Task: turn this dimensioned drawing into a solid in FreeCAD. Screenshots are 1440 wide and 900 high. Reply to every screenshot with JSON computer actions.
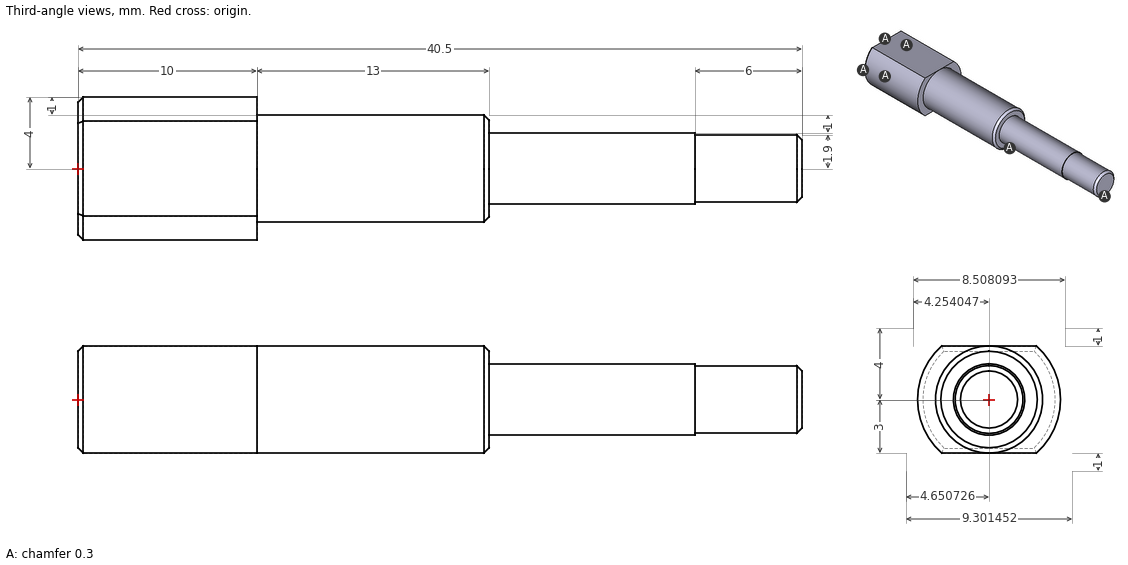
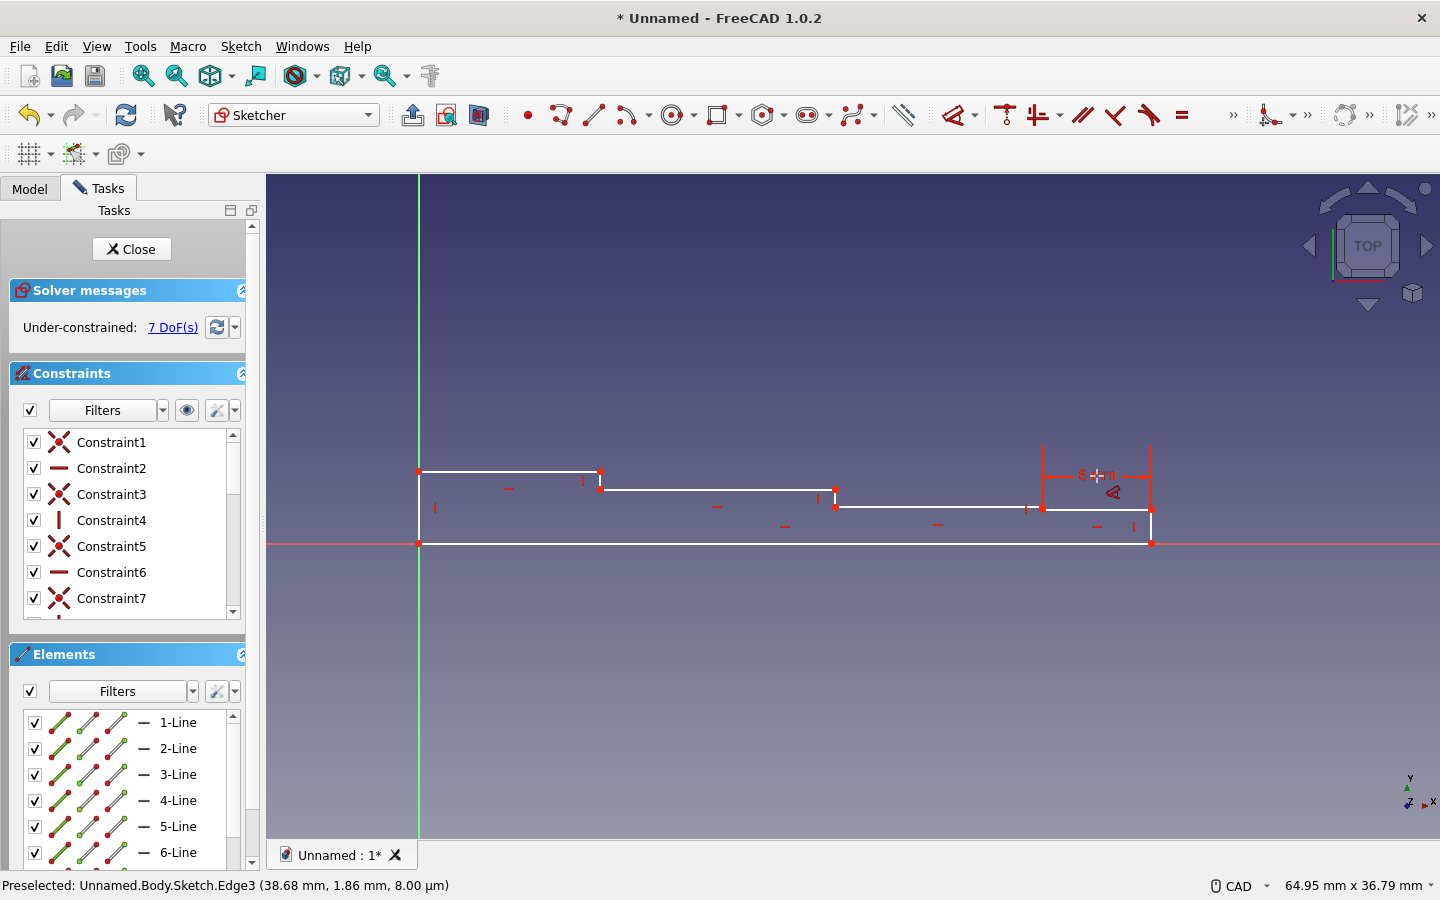
{"action": "scroll", "coordinate": [835, 499], "scroll_direction": "up", "scroll_amount": 4}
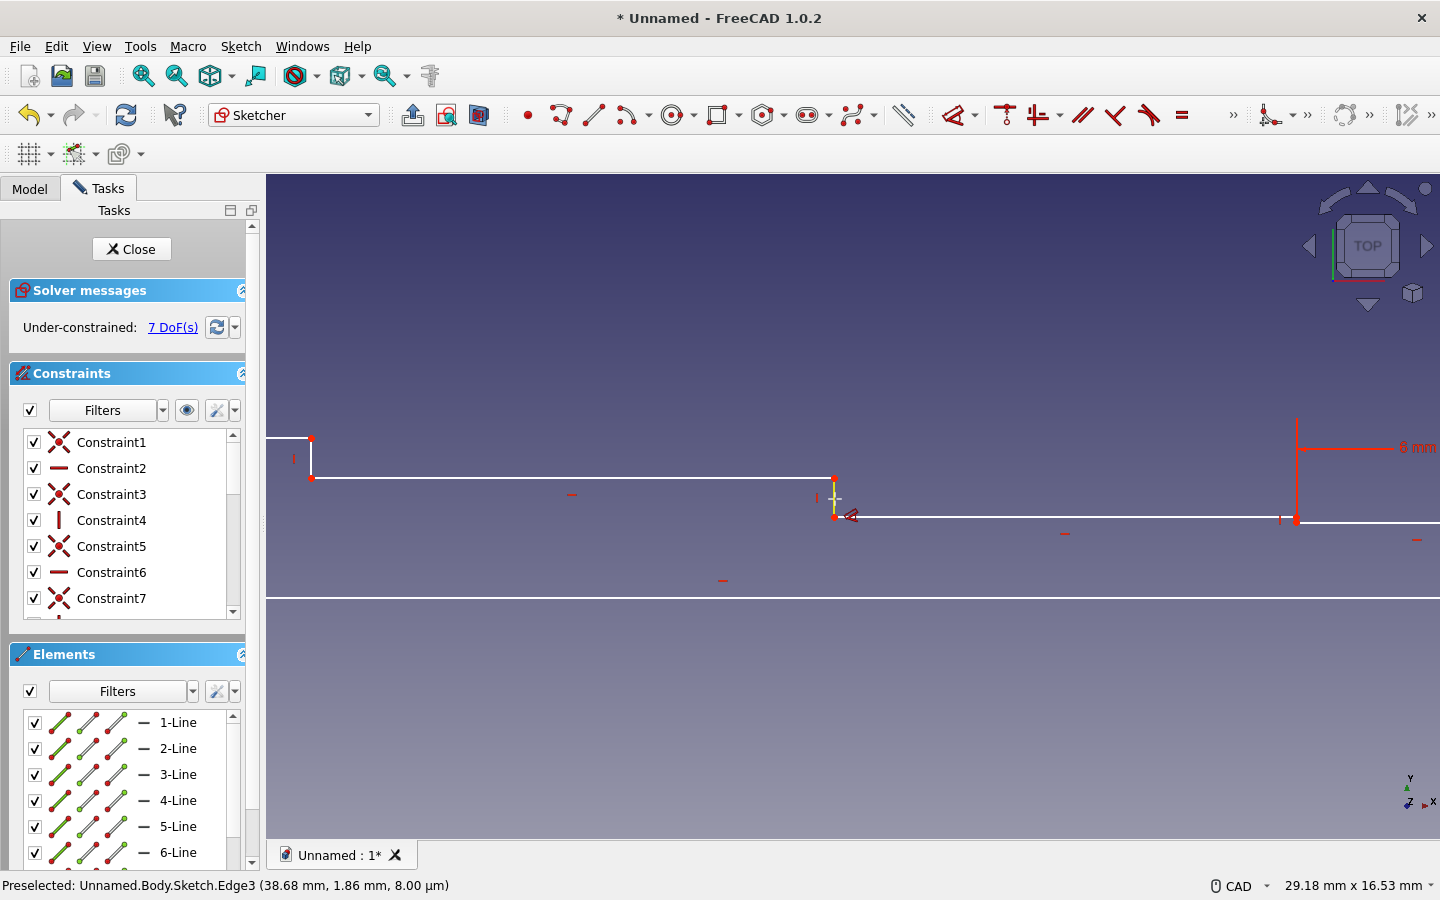
{"action": "left_click", "coordinate": [834, 498]}
{"action": "left_click", "coordinate": [868, 498]}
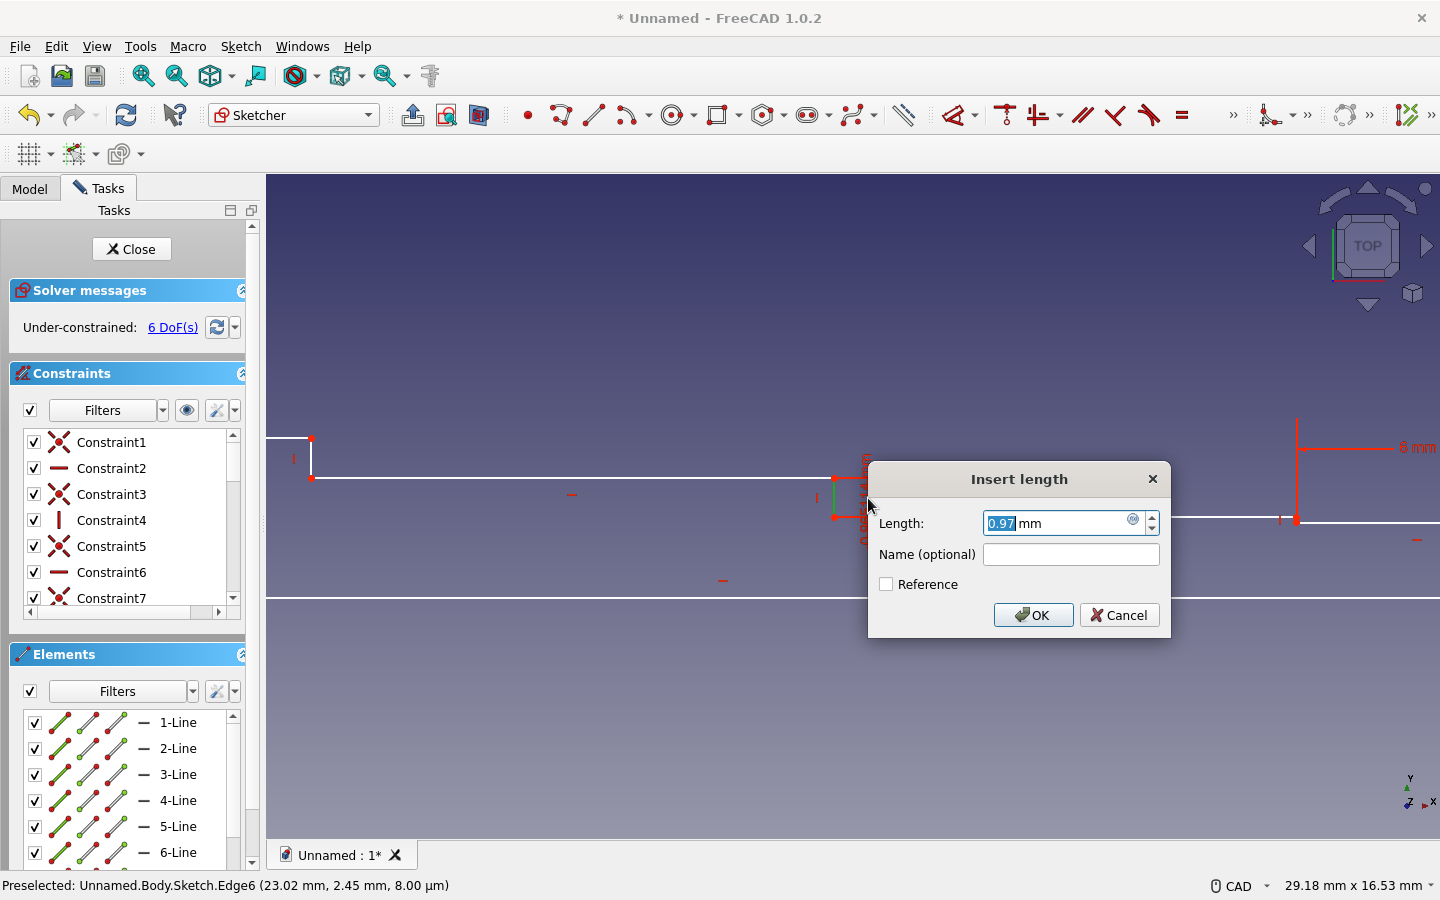
{"action": "type", "text": "1"}
{"action": "key", "text": "Return"}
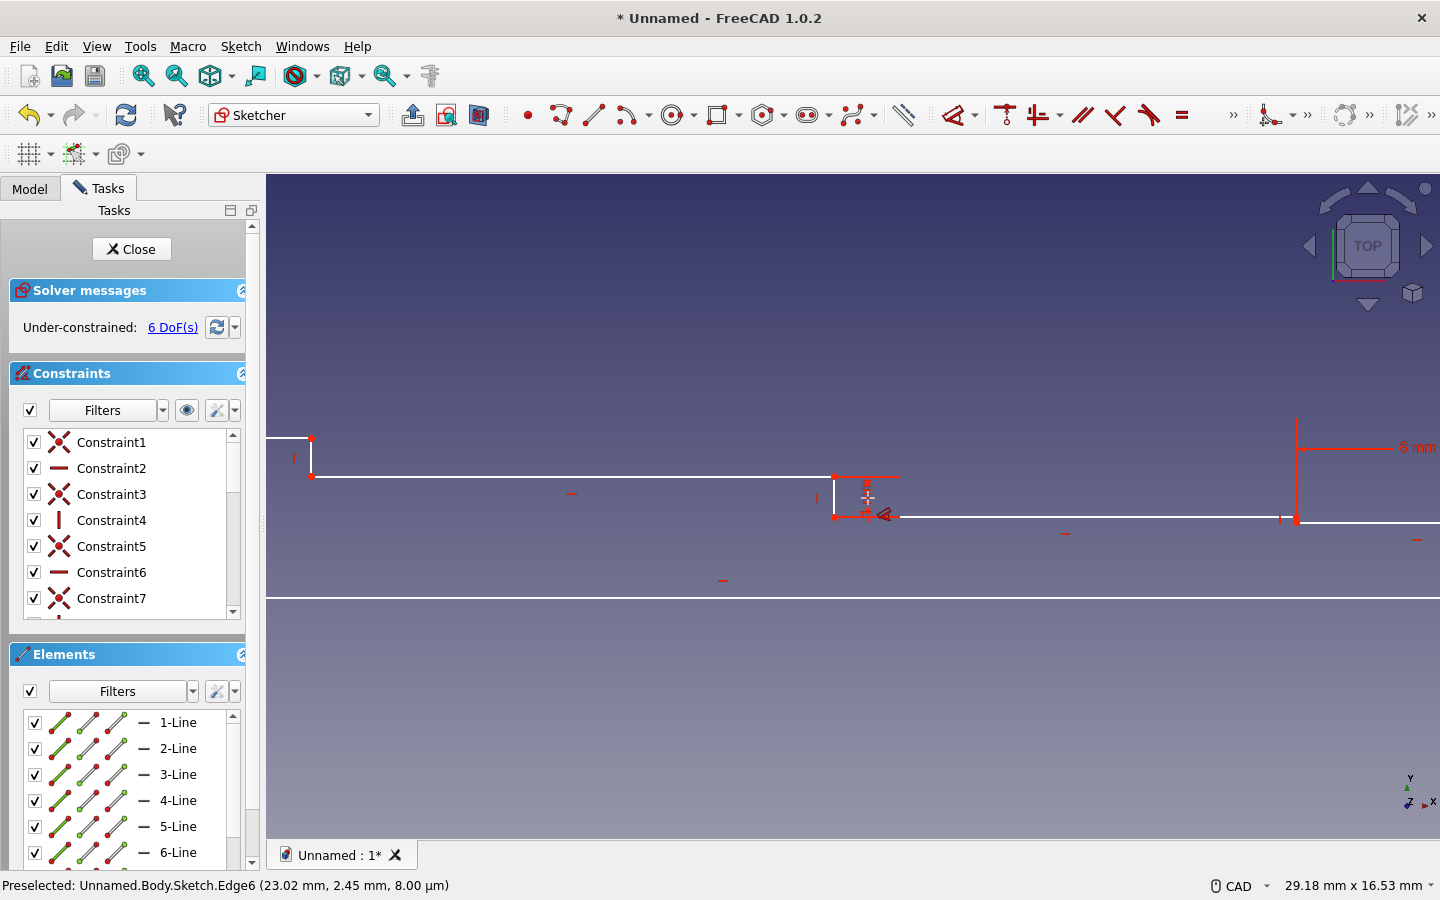
{"action": "left_click", "coordinate": [311, 465]}
{"action": "left_click", "coordinate": [345, 458]}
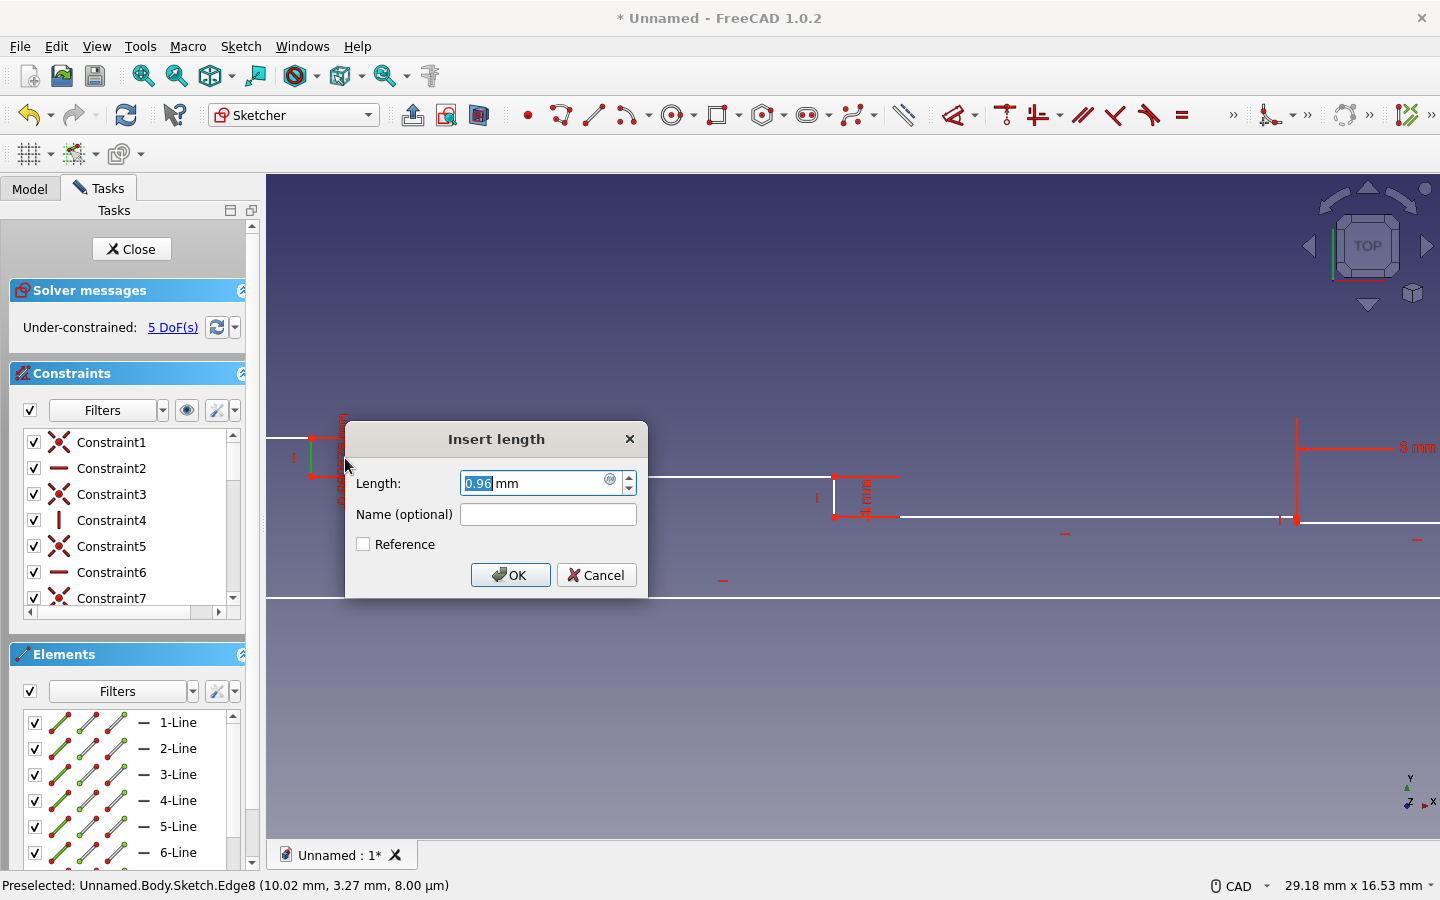
{"action": "type", "text": "1"}
{"action": "key", "text": "Return"}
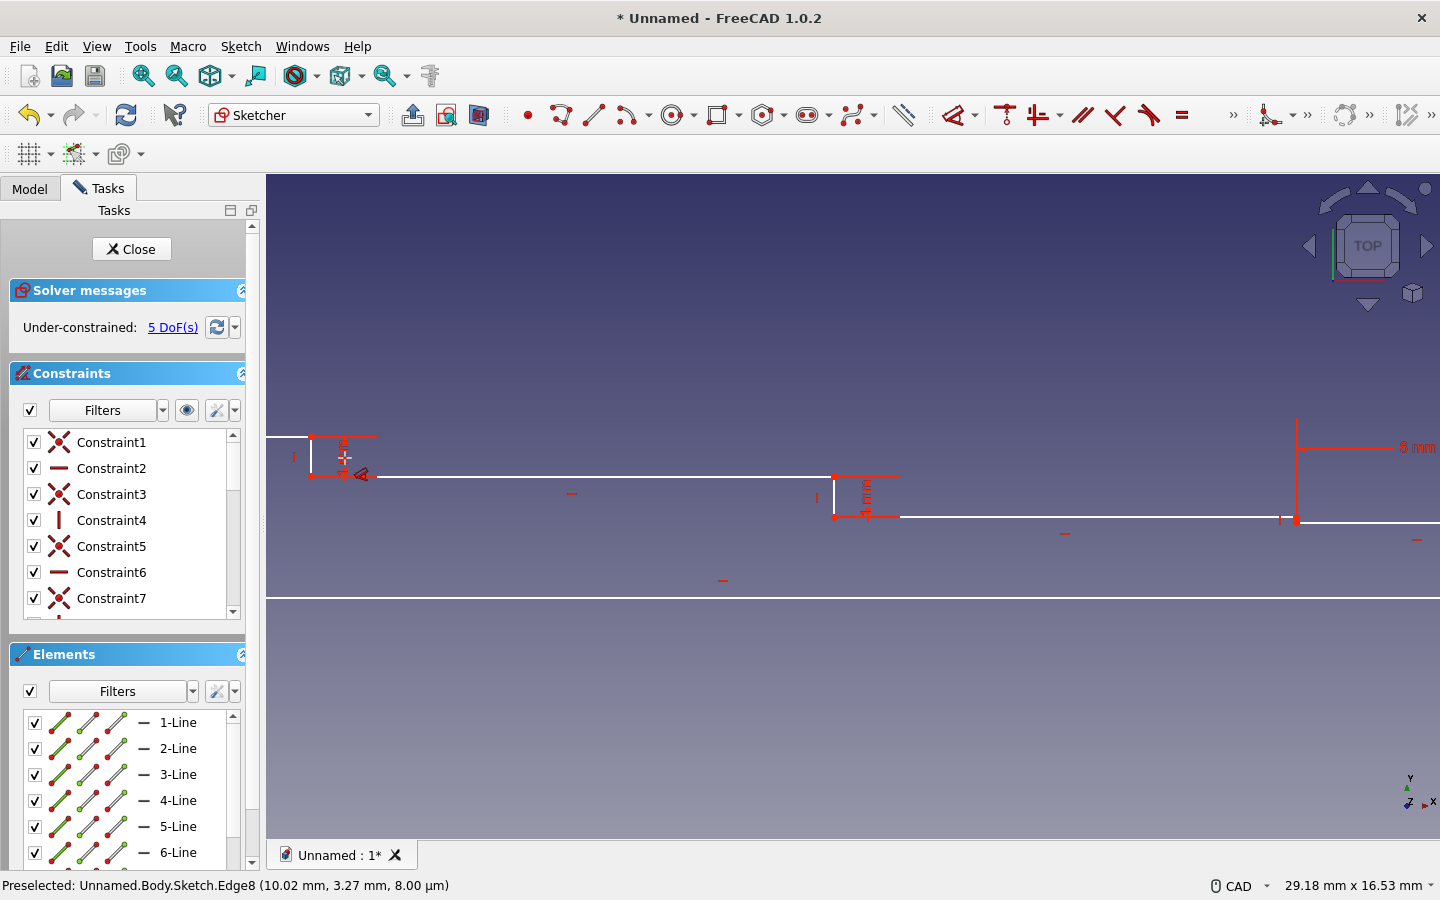
{"action": "scroll", "coordinate": [835, 498], "scroll_direction": "down", "scroll_amount": 4}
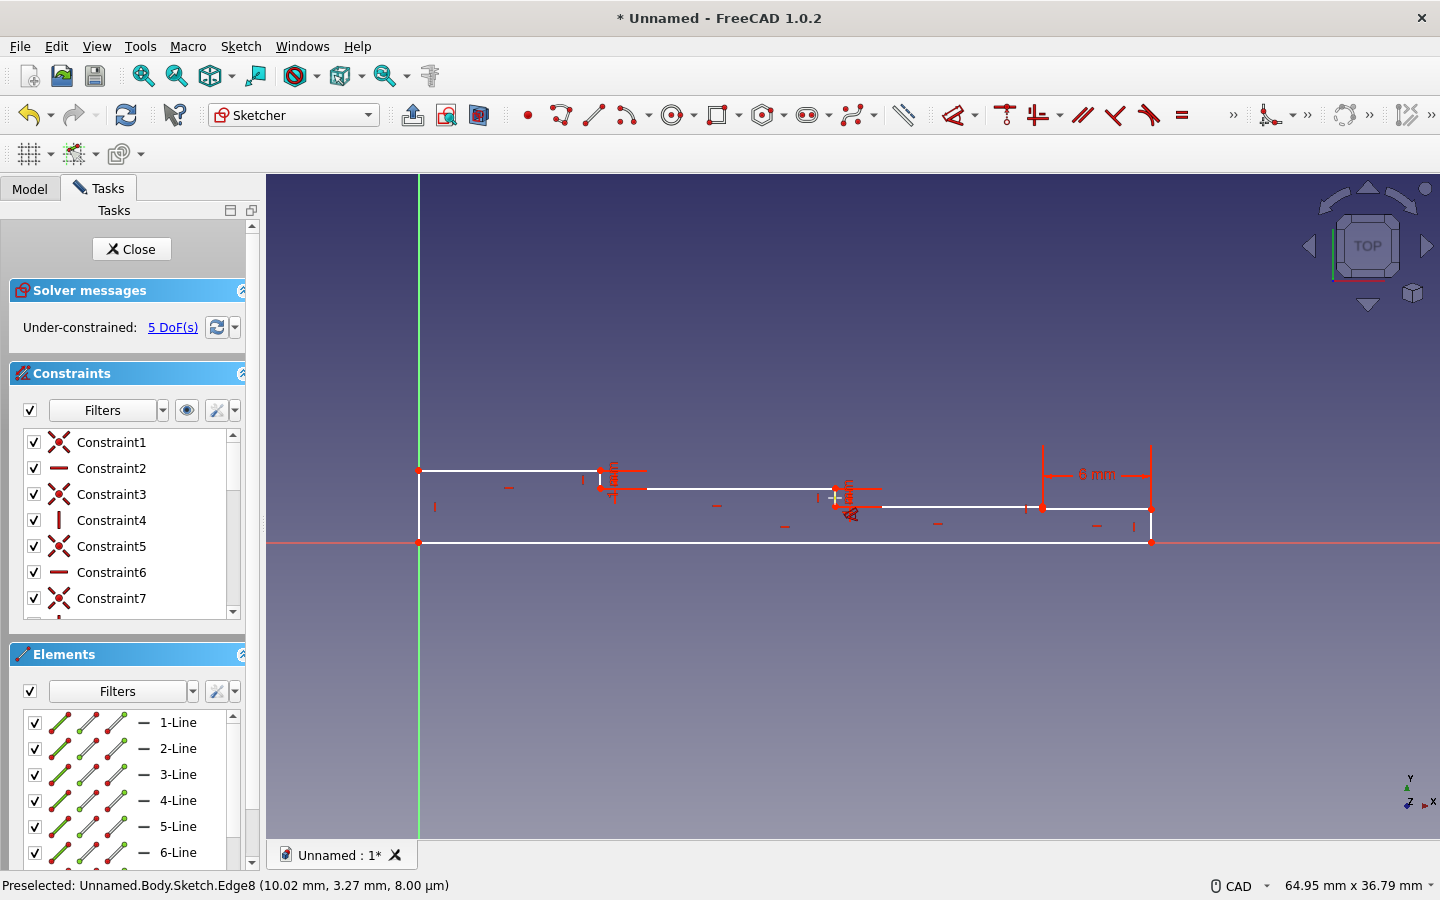
{"action": "left_click", "coordinate": [419, 492]}
{"action": "left_click", "coordinate": [385, 507]}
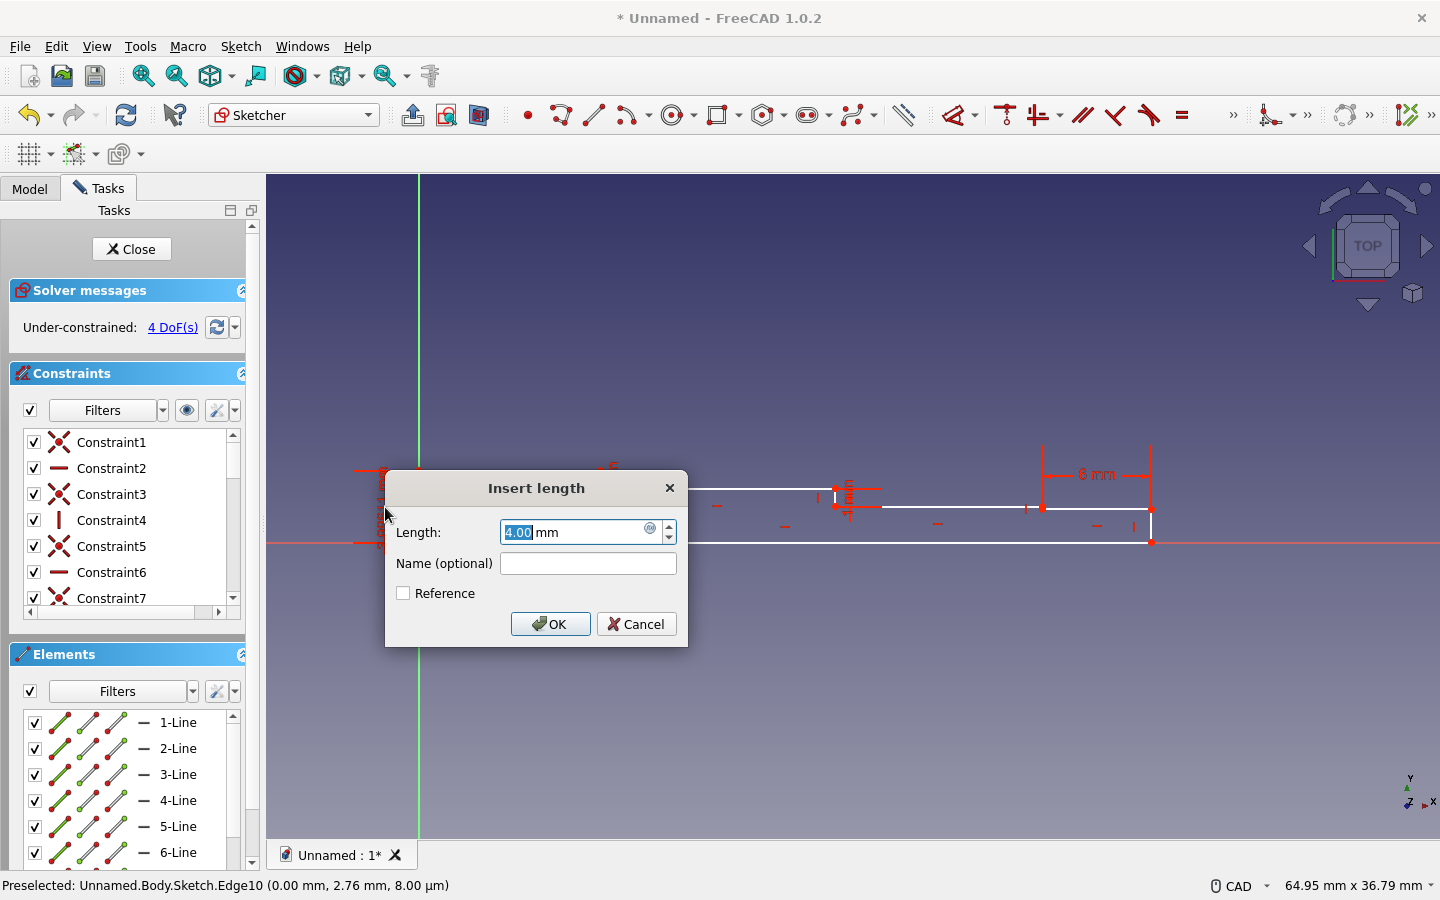
{"action": "type", "text": "4"}
{"action": "key", "text": "Return"}